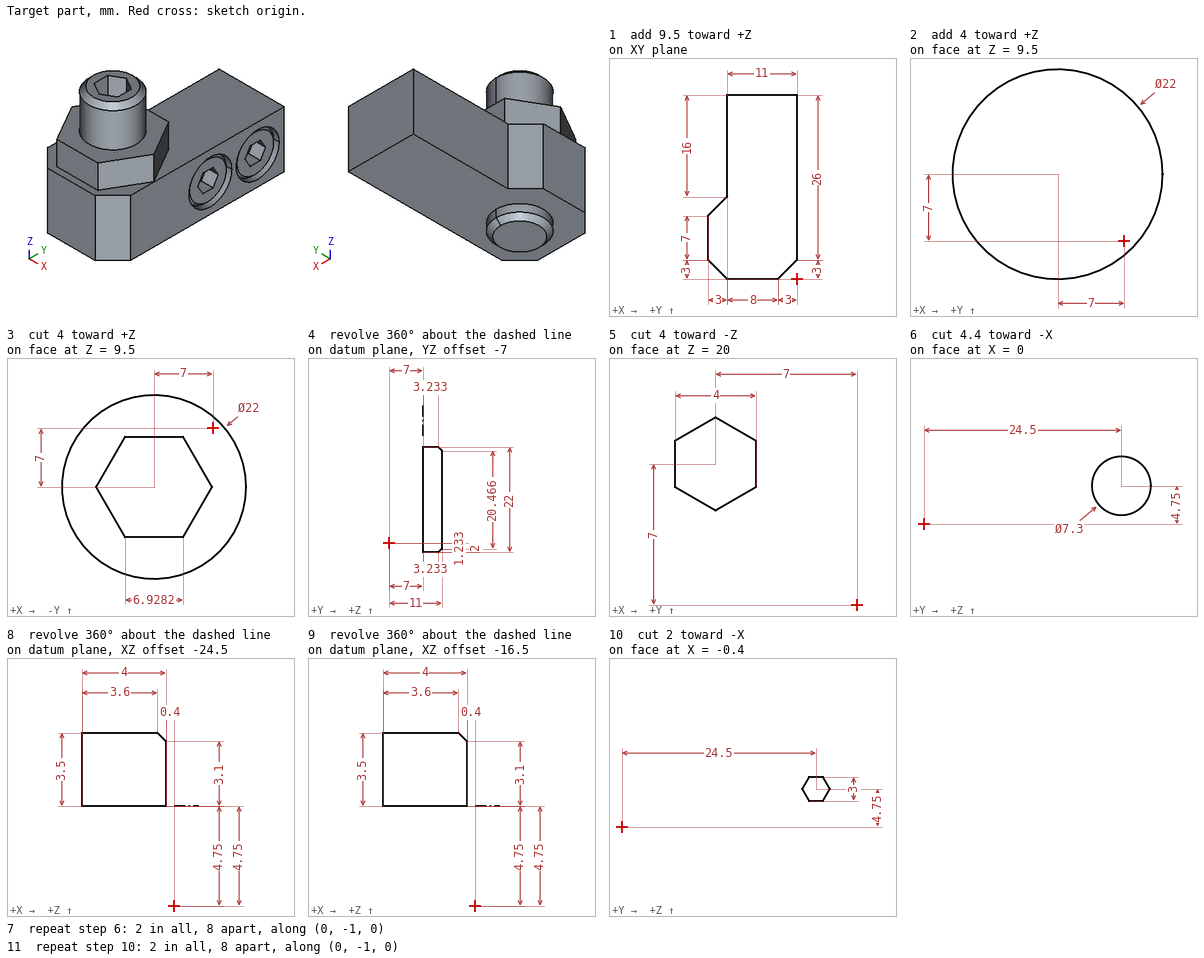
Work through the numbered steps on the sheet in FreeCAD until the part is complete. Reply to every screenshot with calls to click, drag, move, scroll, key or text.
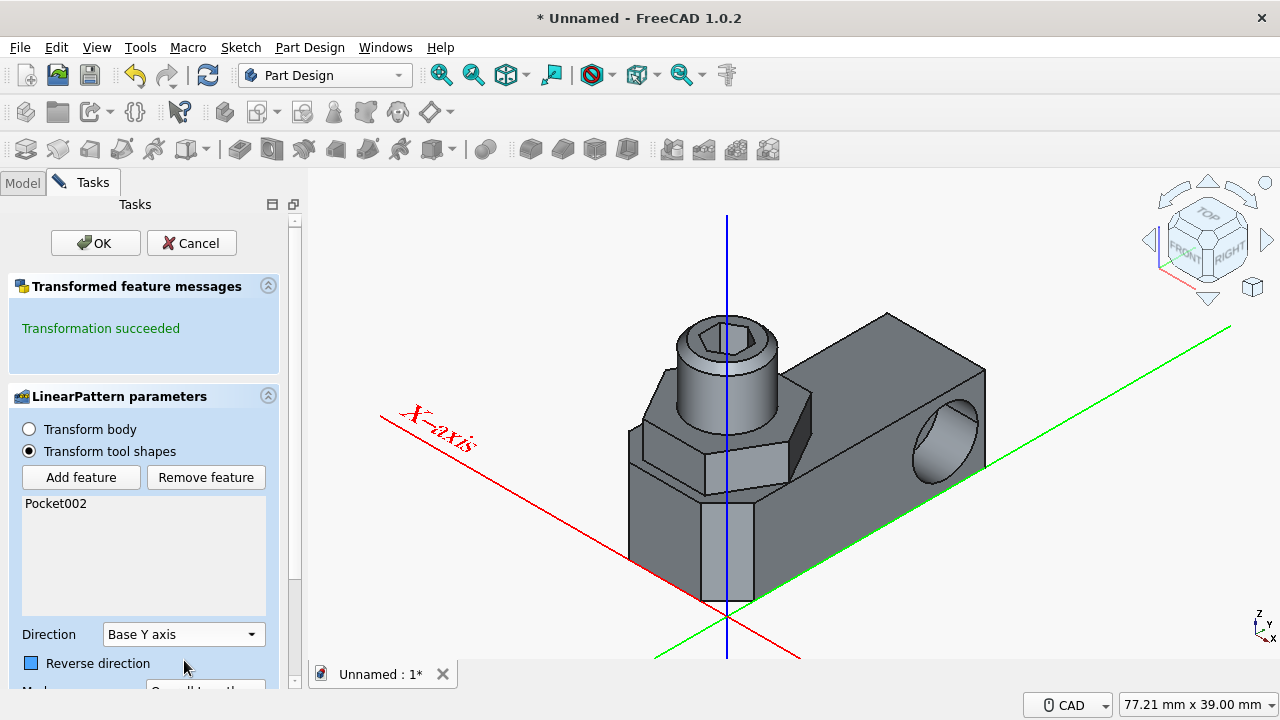
scroll(295, 451, down, 2)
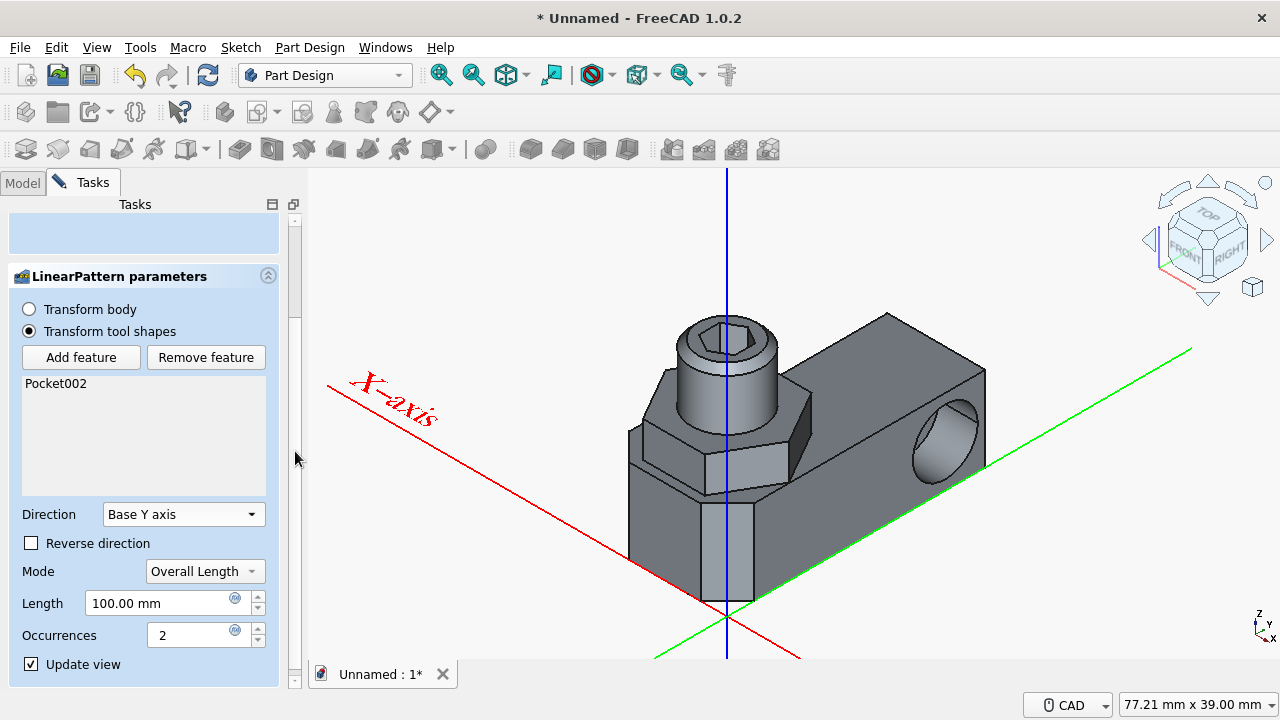
click(206, 572)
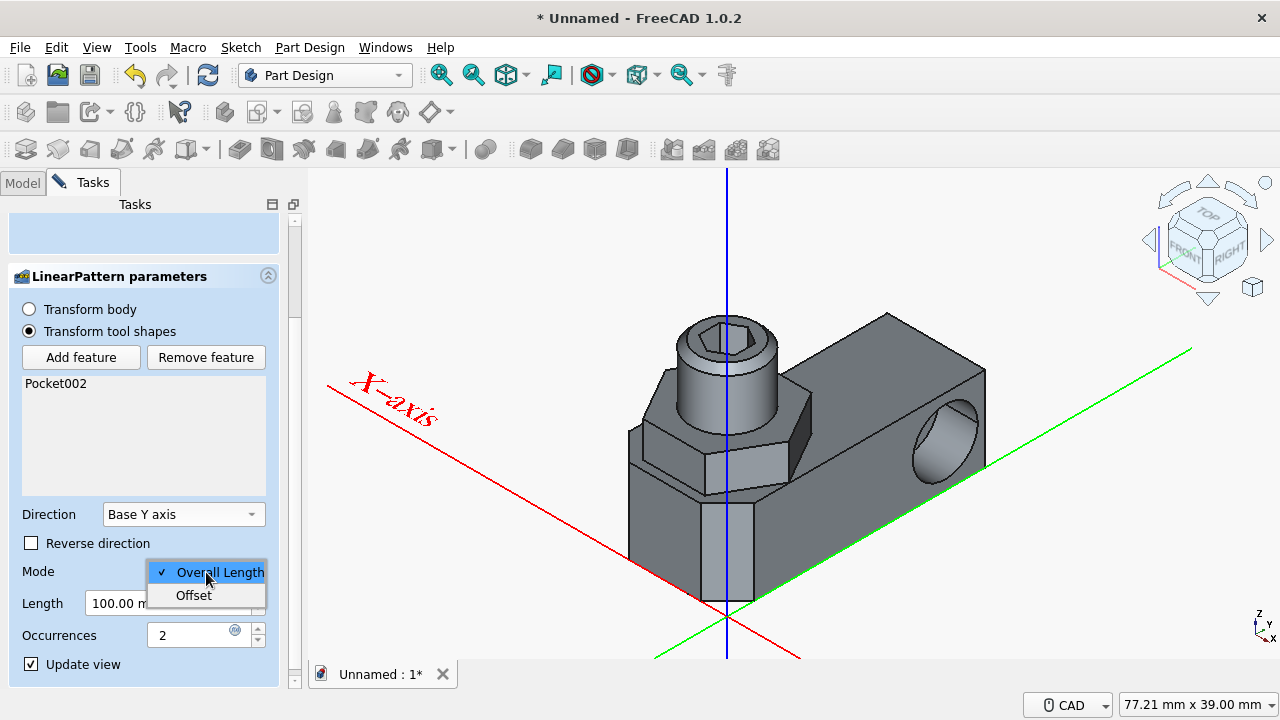
click(206, 596)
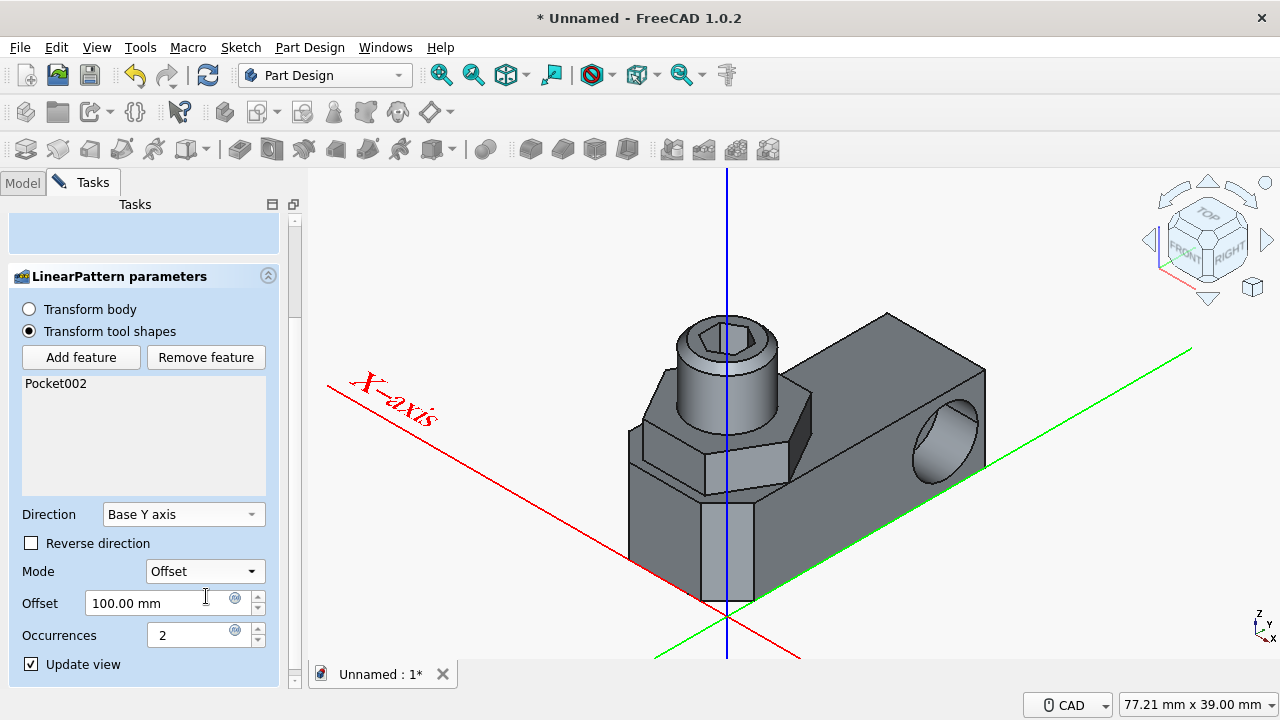
triple_click(168, 603)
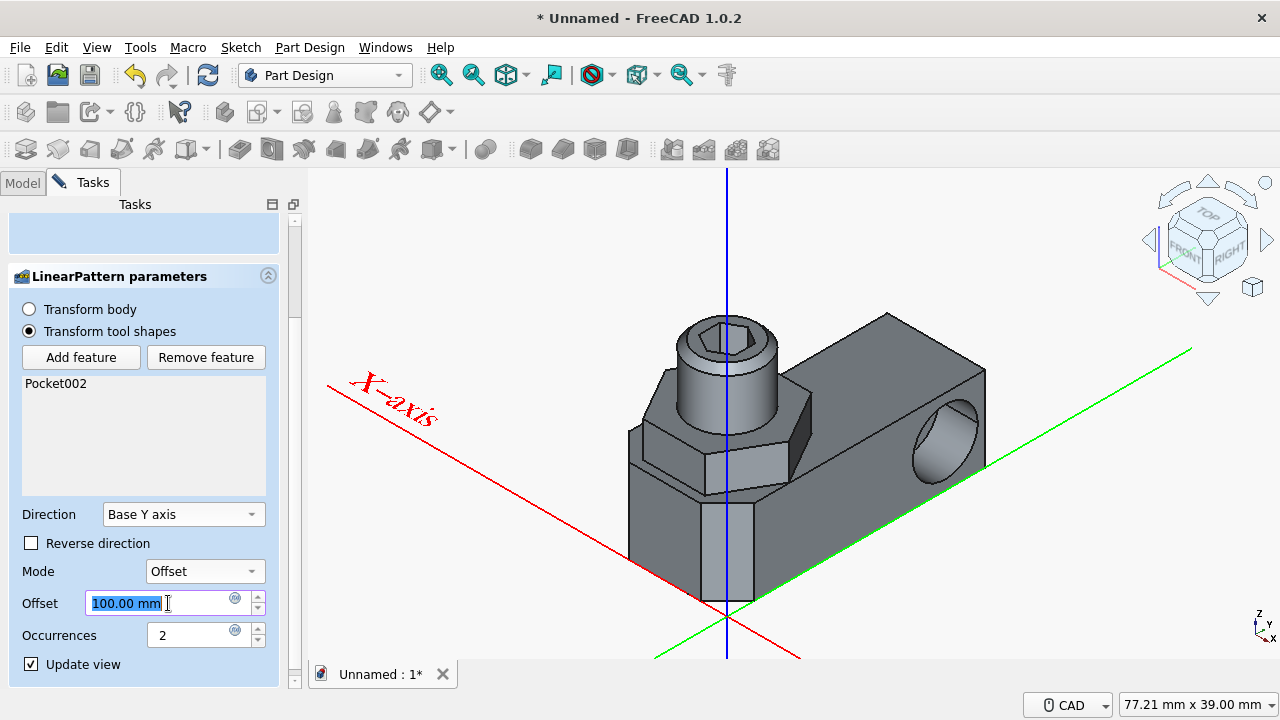
text(8)
key(Tab)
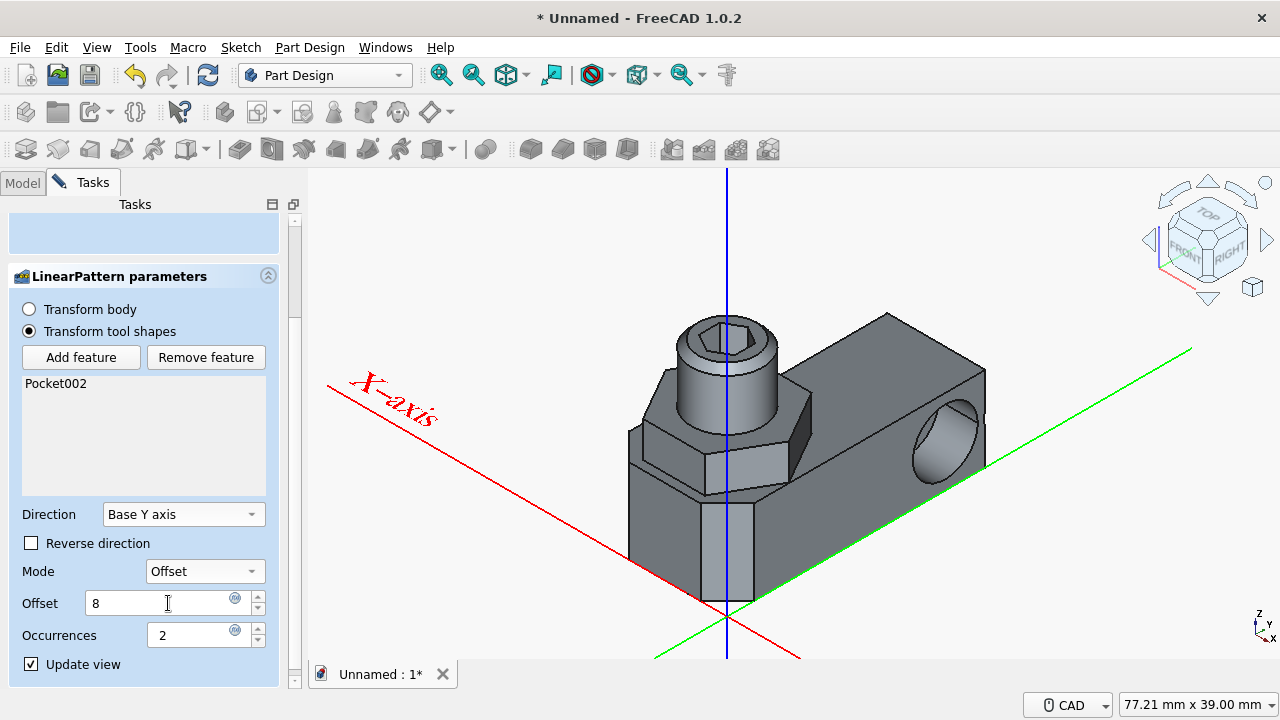
triple_click(198, 635)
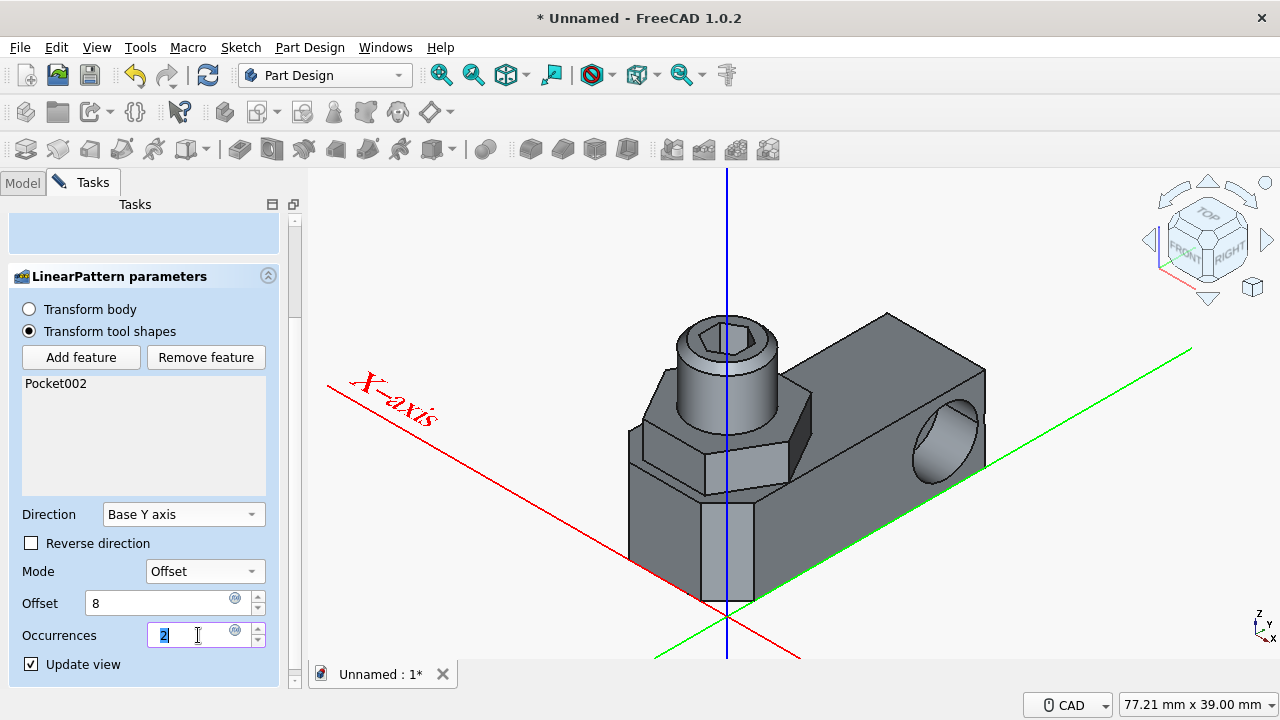
text(2)
key(Tab)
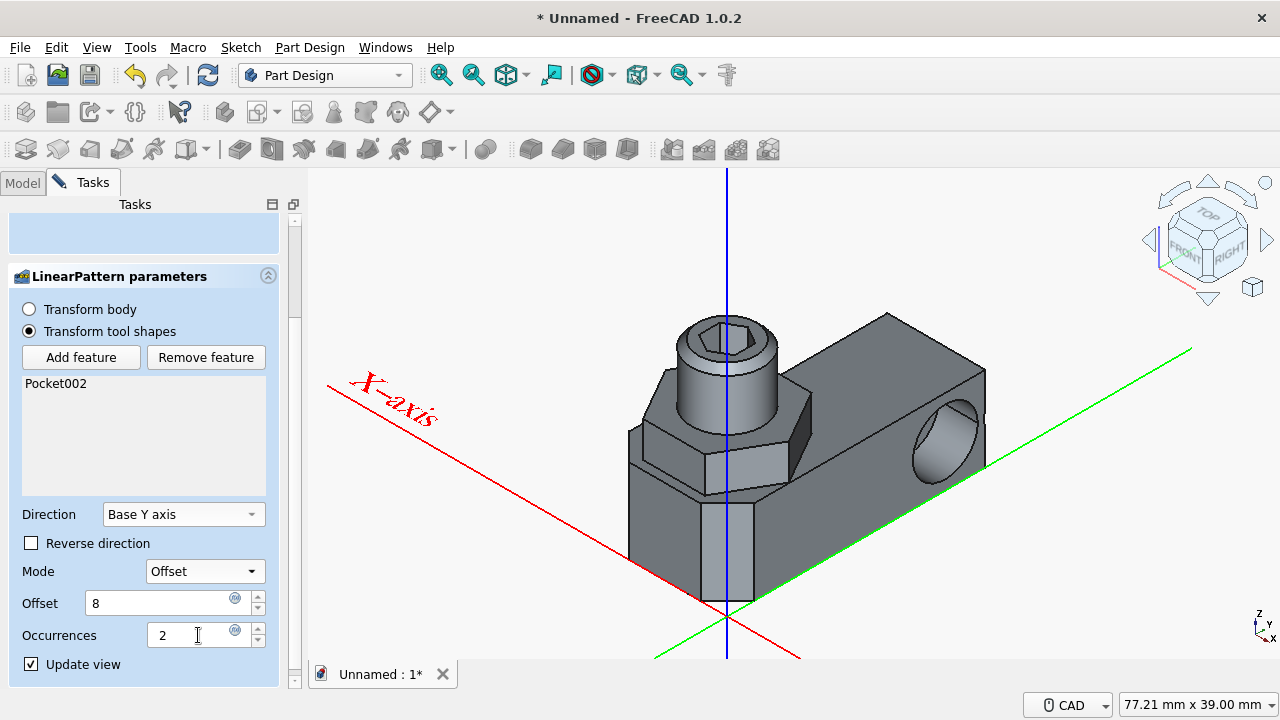
click(30, 543)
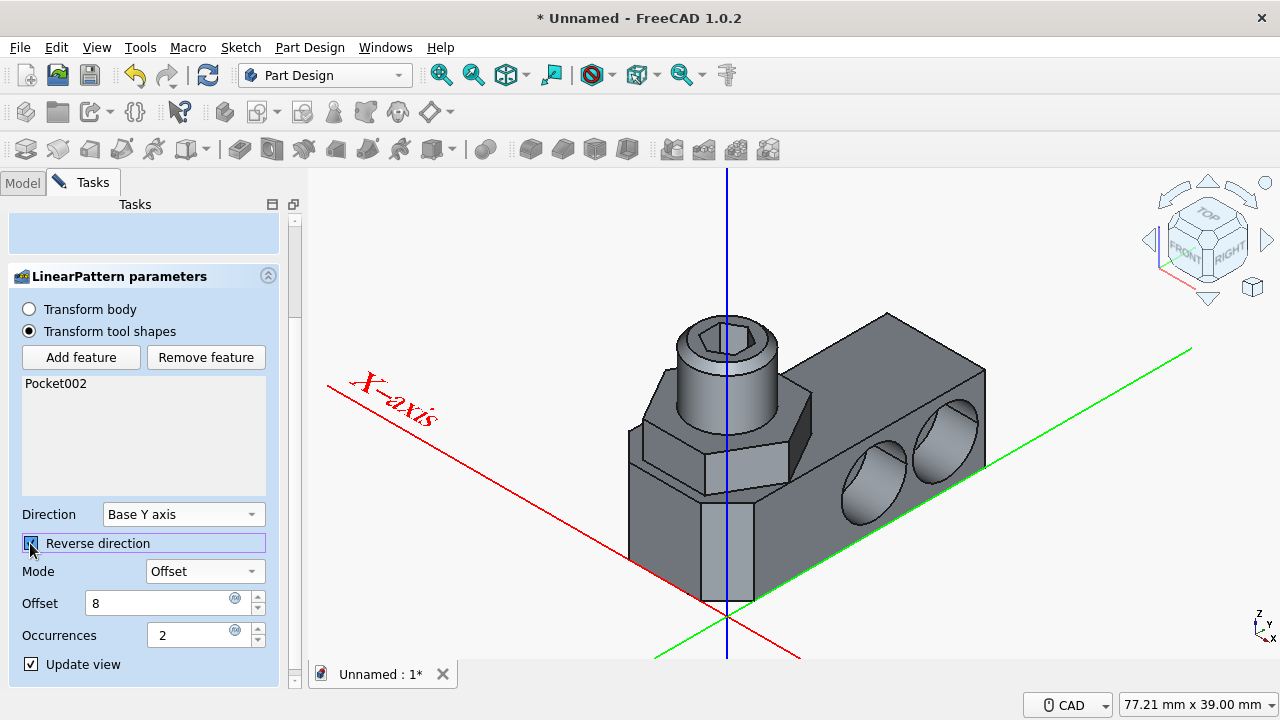
scroll(295, 451, up, 3)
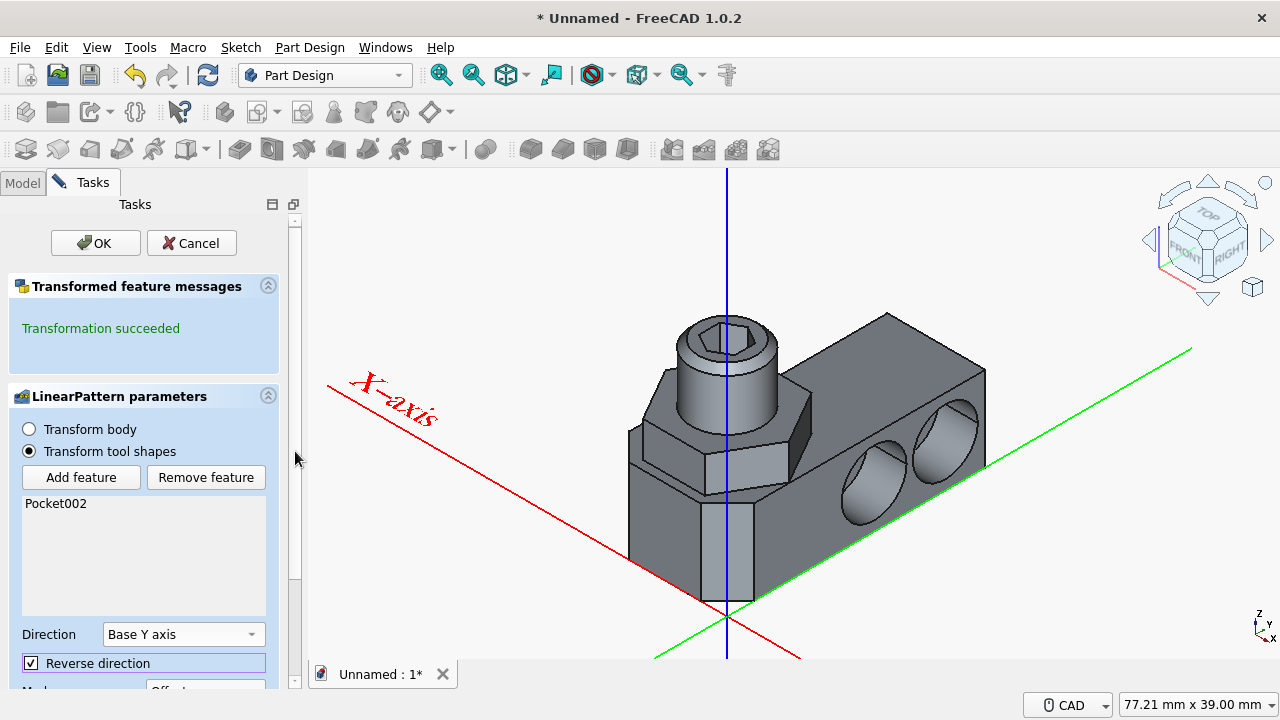
click(96, 243)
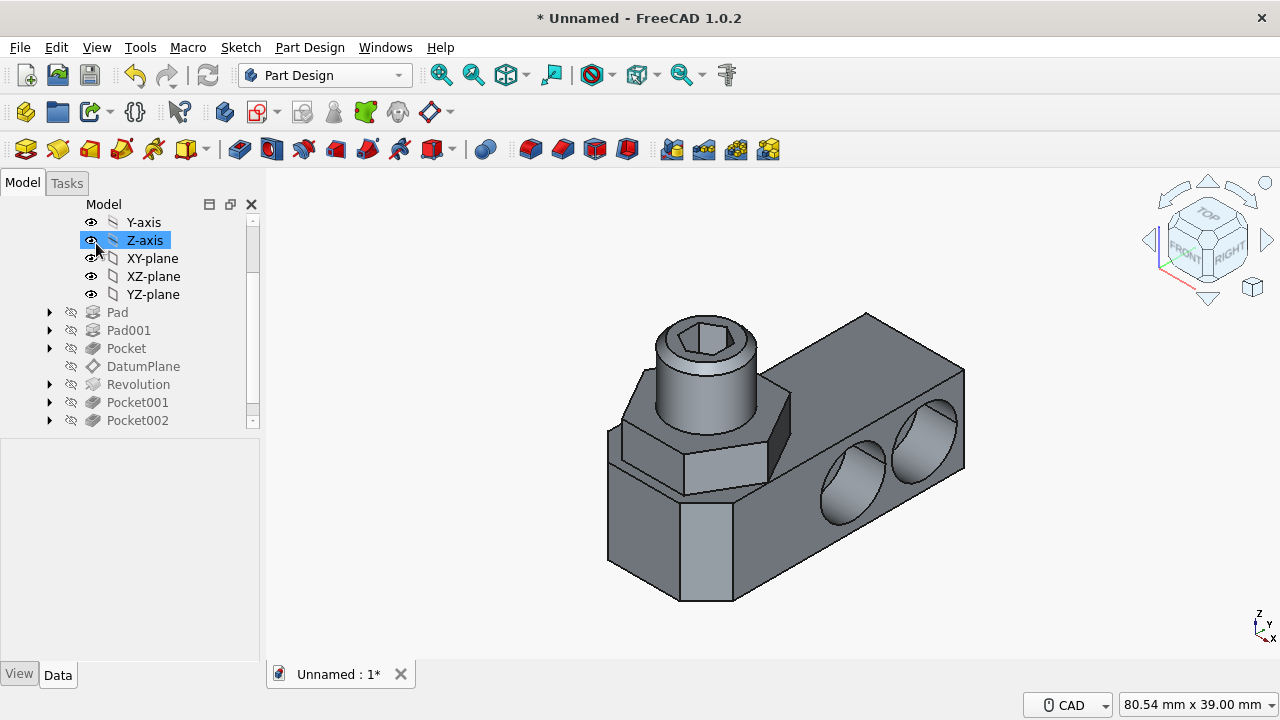
scroll(160, 326, down, 3)